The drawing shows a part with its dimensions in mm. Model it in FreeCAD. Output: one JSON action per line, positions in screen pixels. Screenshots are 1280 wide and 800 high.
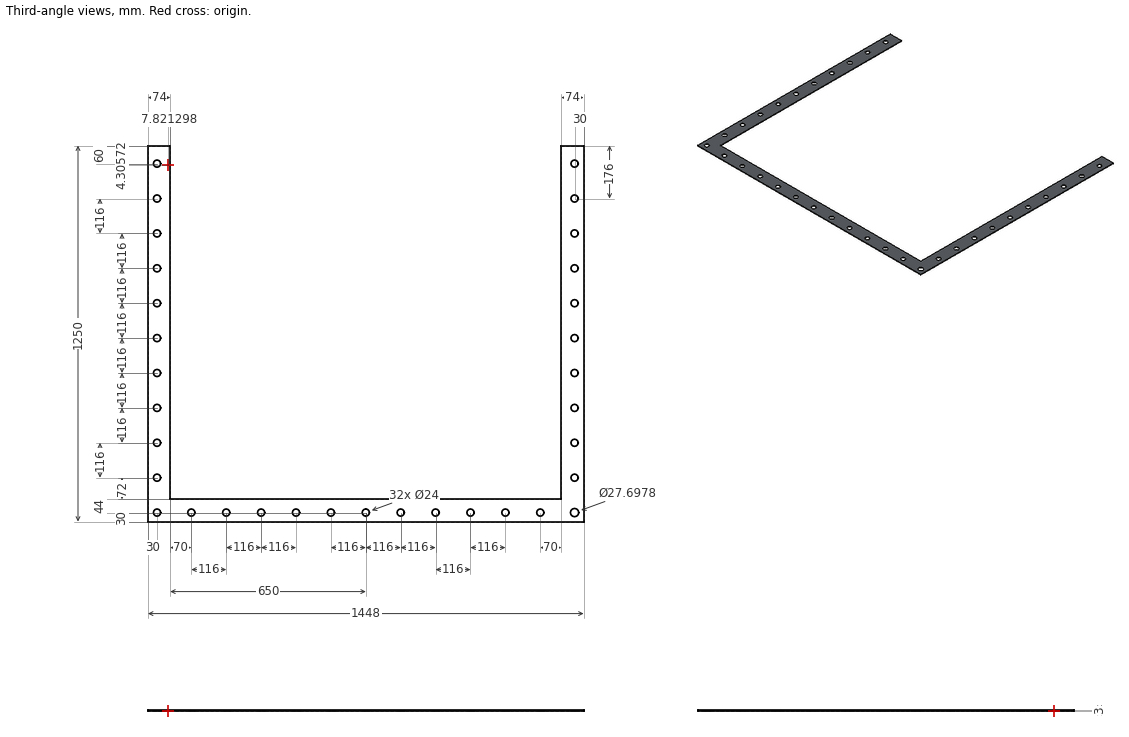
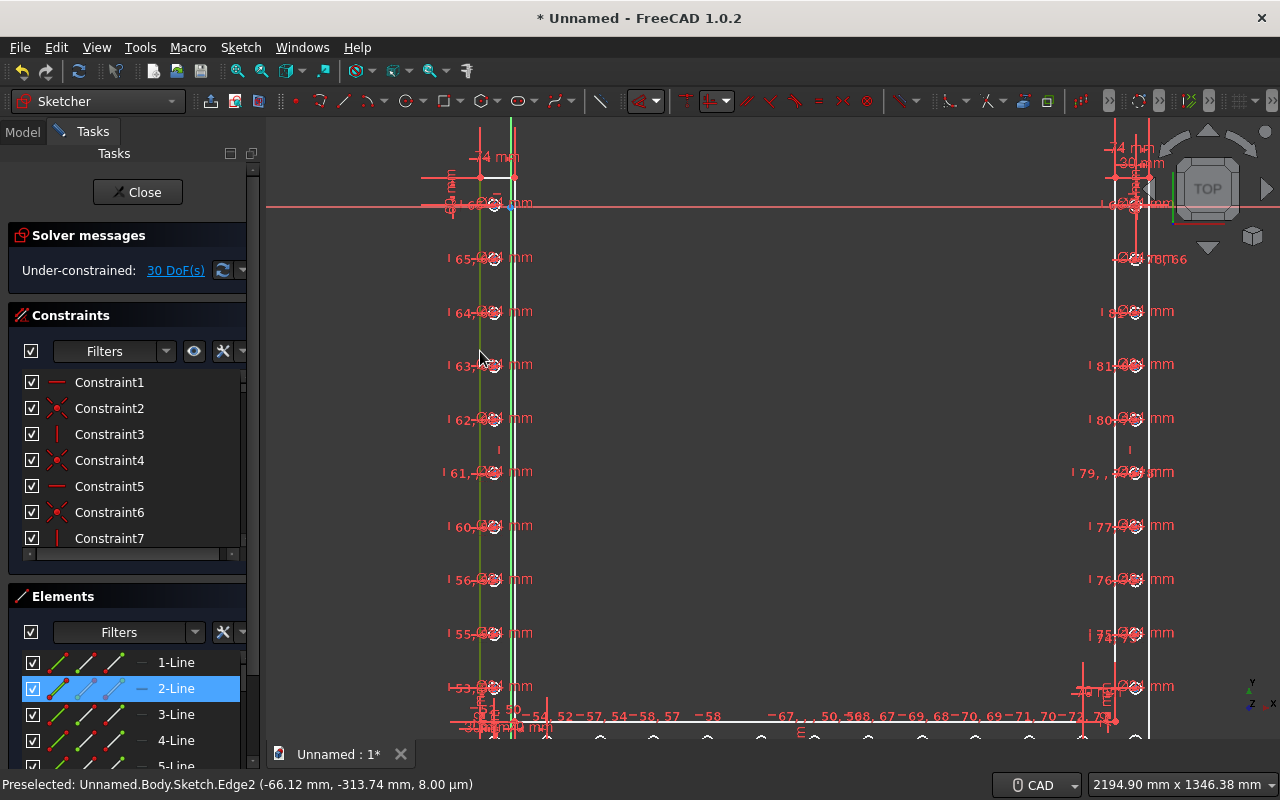
{"action": "left_click", "coordinate": [658, 102]}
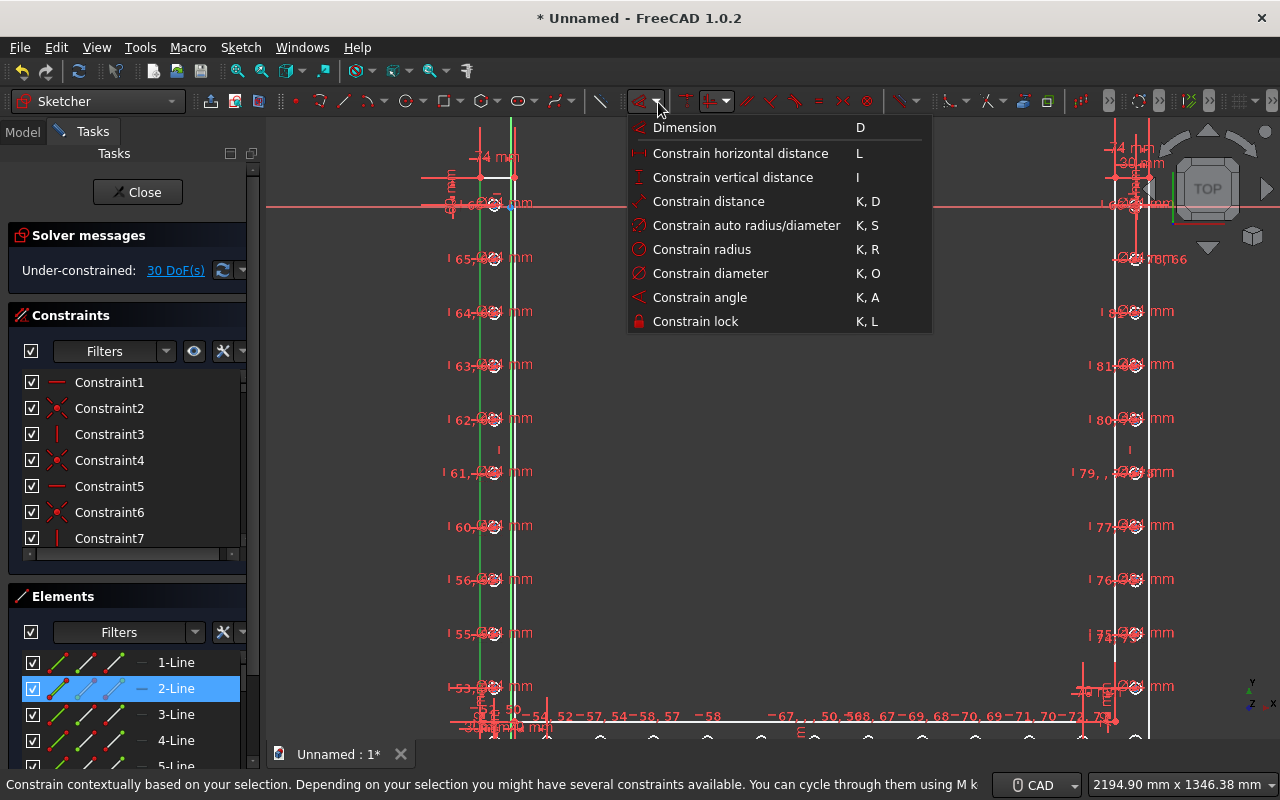
{"action": "left_click", "coordinate": [780, 177]}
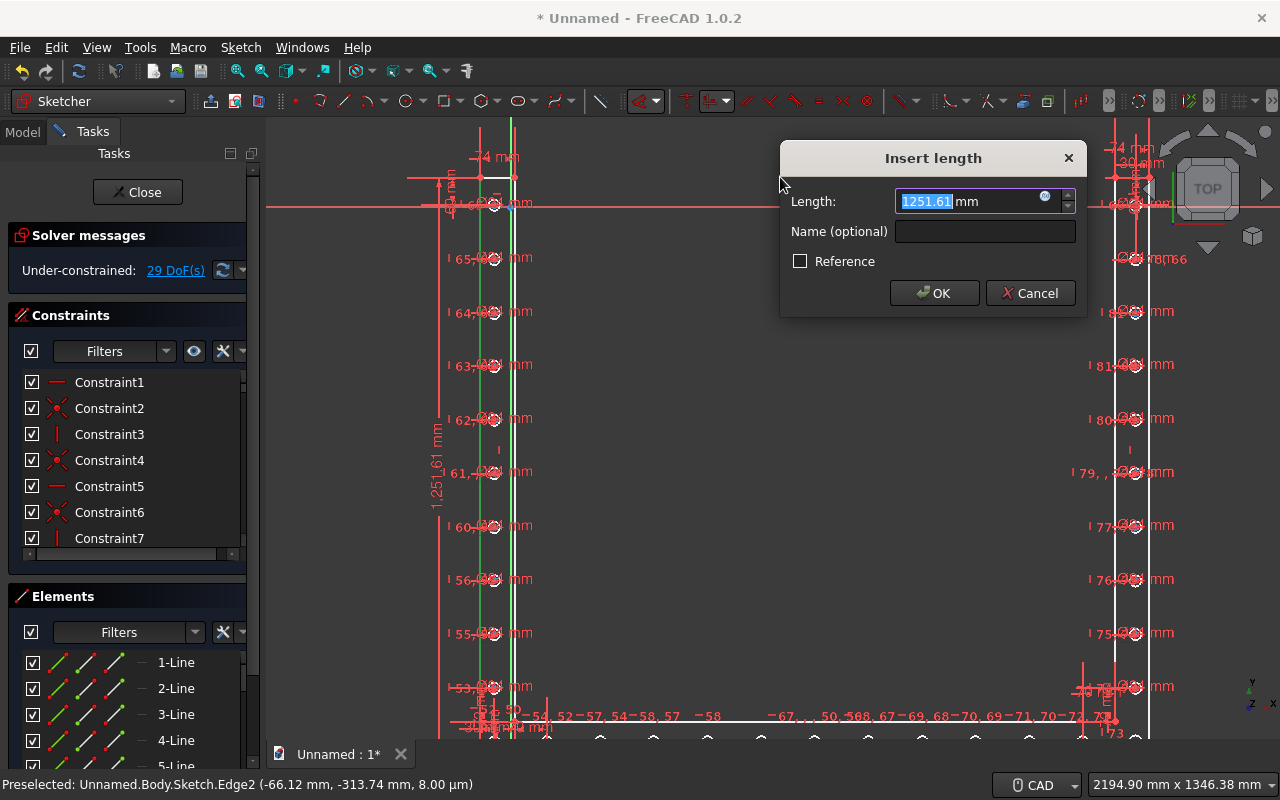
{"action": "type", "text": "1250"}
{"action": "key", "text": "Return"}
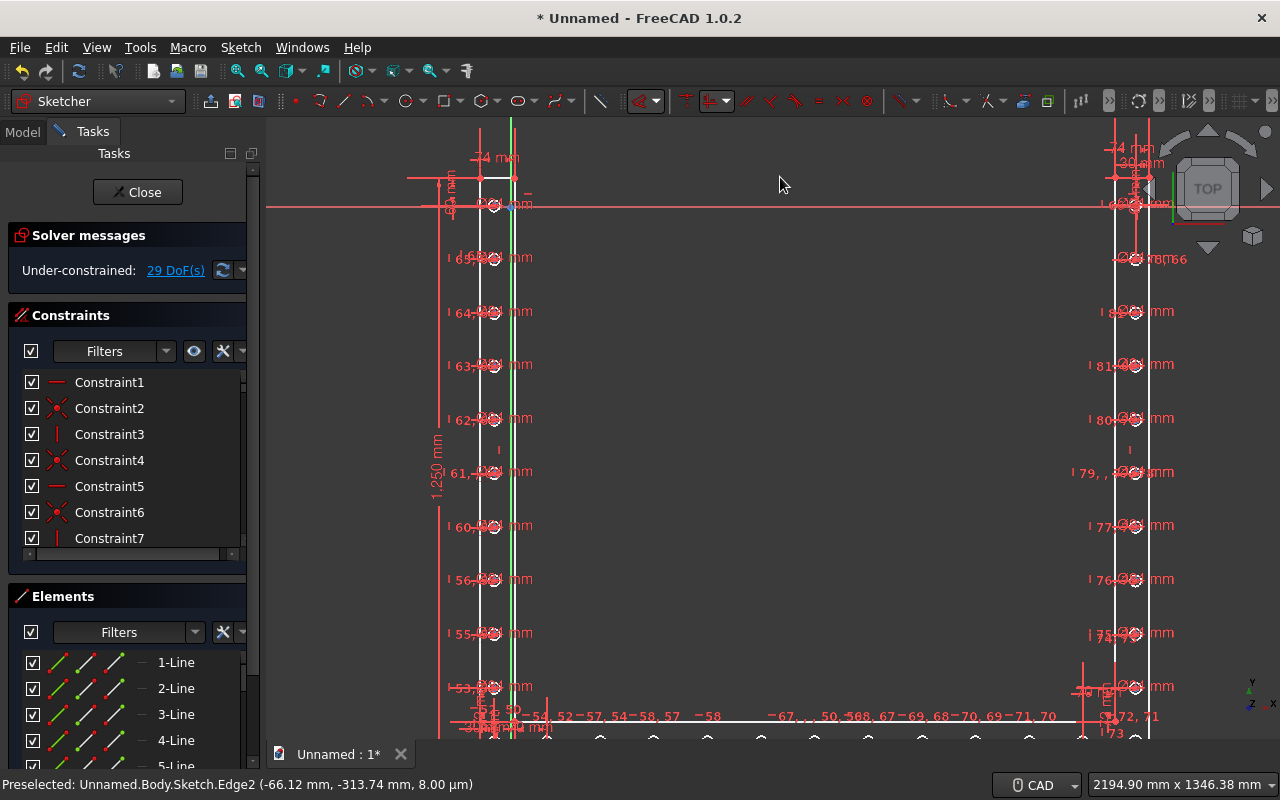
{"action": "scroll", "coordinate": [480, 351], "scroll_direction": "down", "scroll_amount": 2}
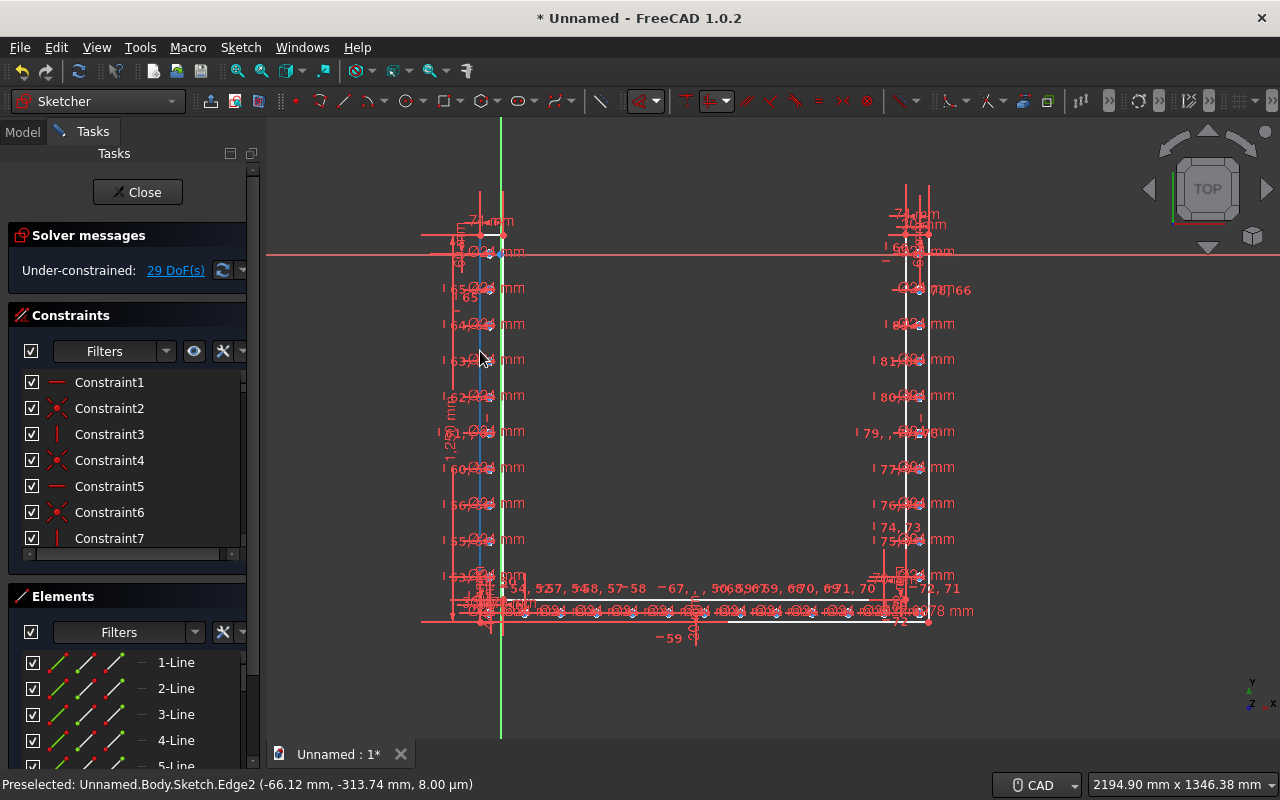
{"action": "left_click", "coordinate": [615, 622]}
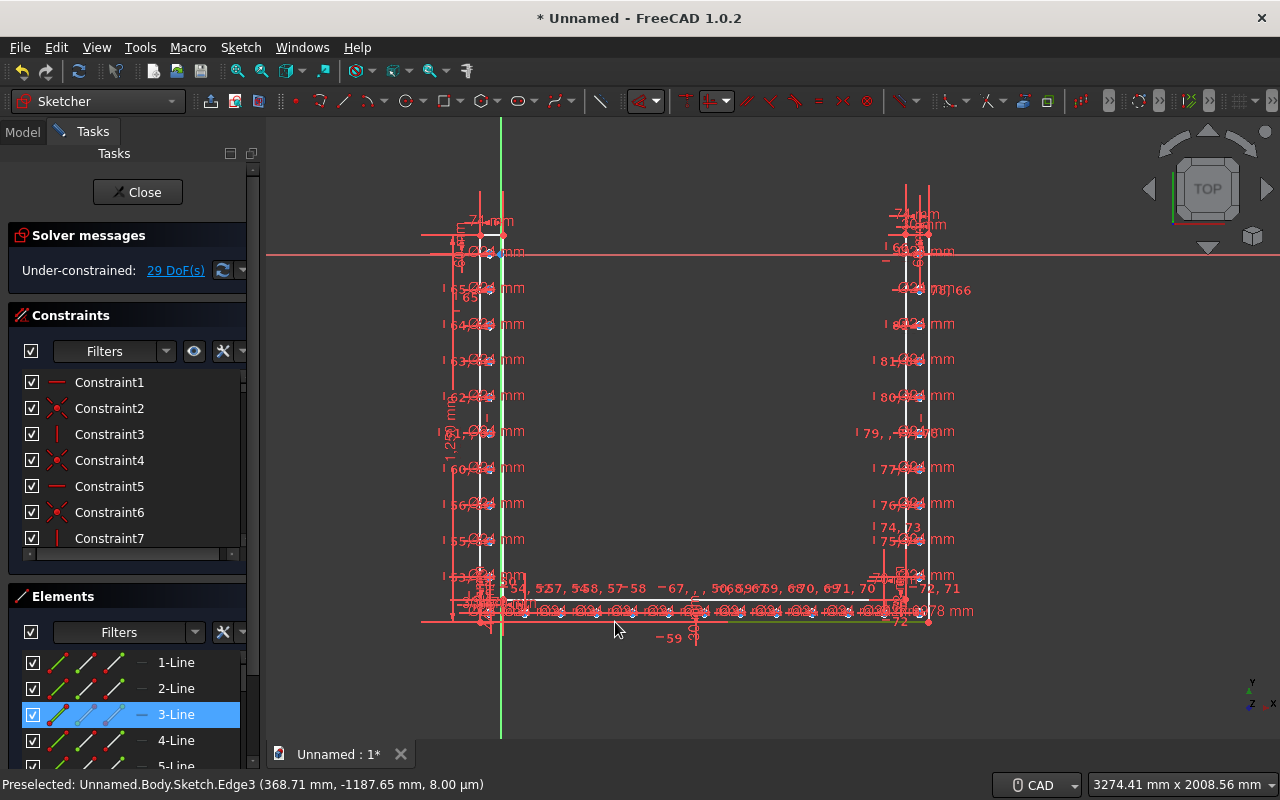
{"action": "left_click", "coordinate": [658, 102]}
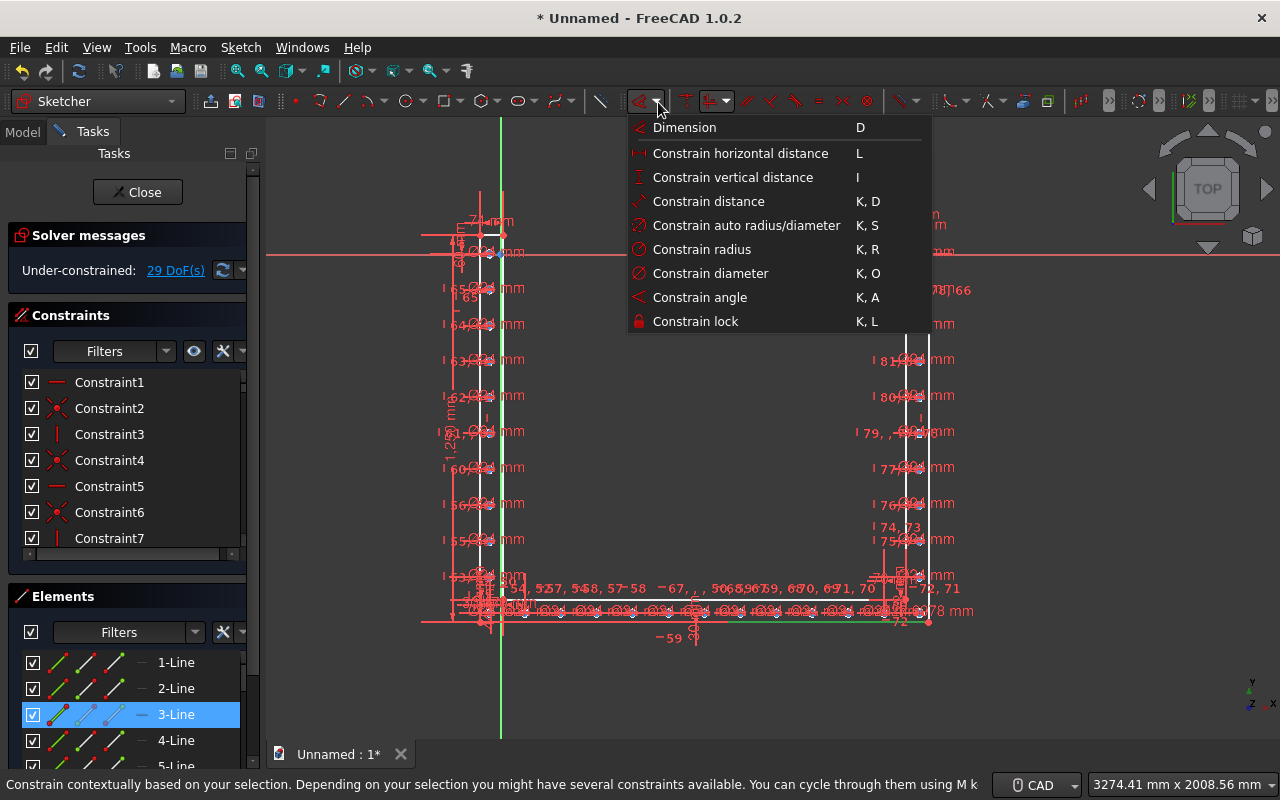
{"action": "left_click", "coordinate": [780, 153]}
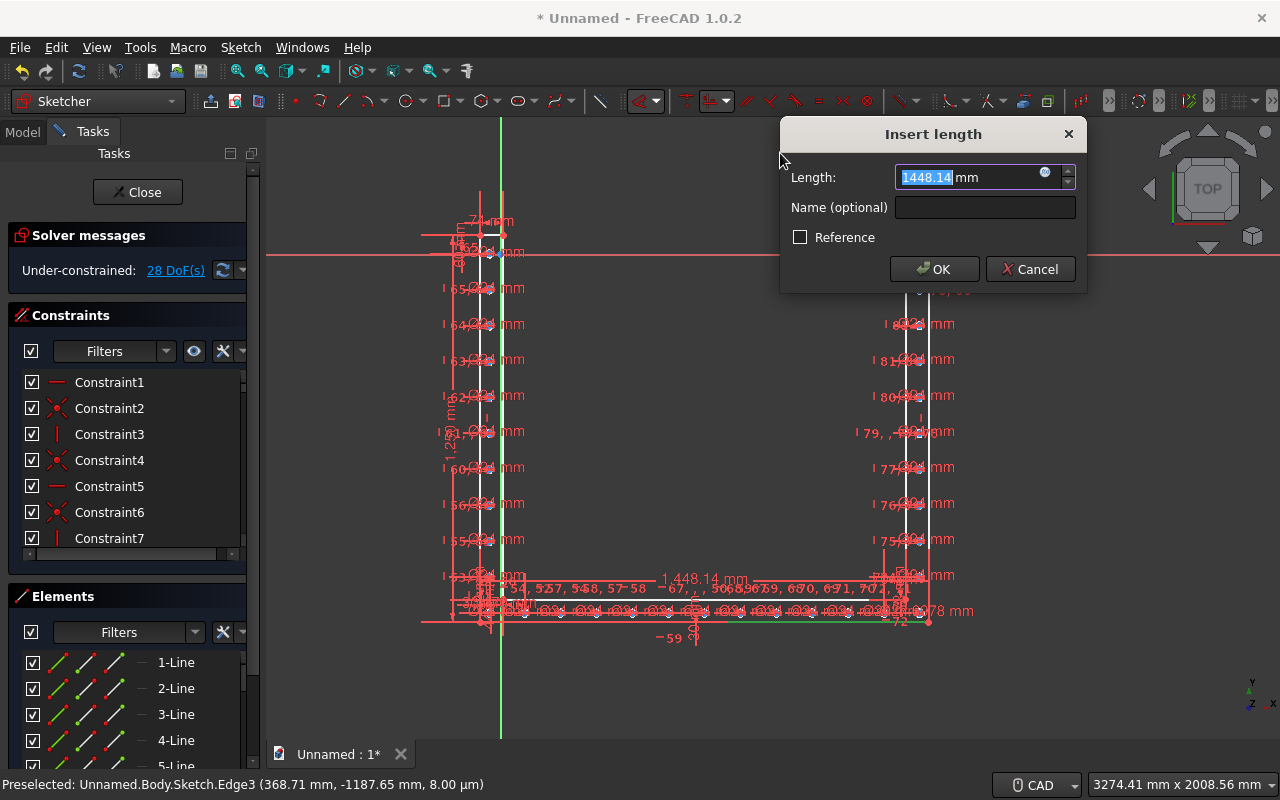
{"action": "type", "text": "1448"}
{"action": "key", "text": "Return"}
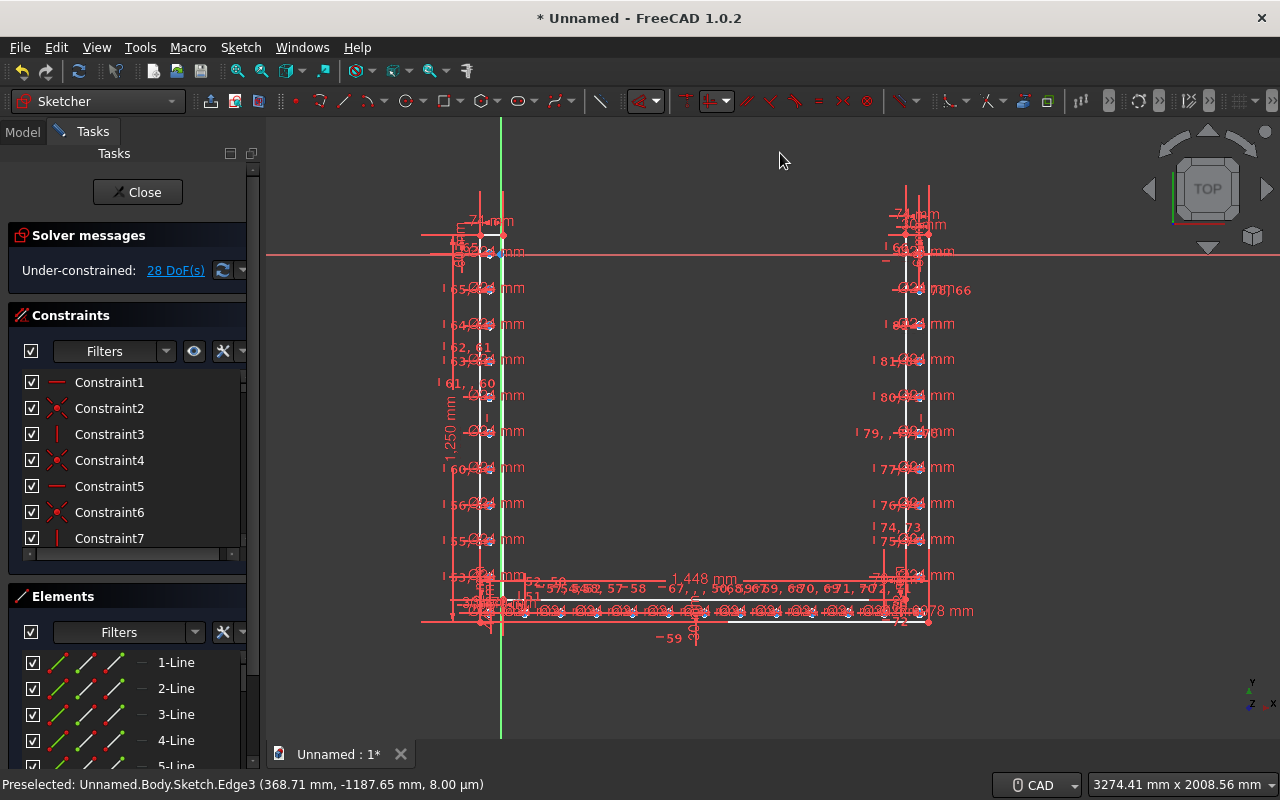
{"action": "scroll", "coordinate": [929, 351], "scroll_direction": "up", "scroll_amount": 2}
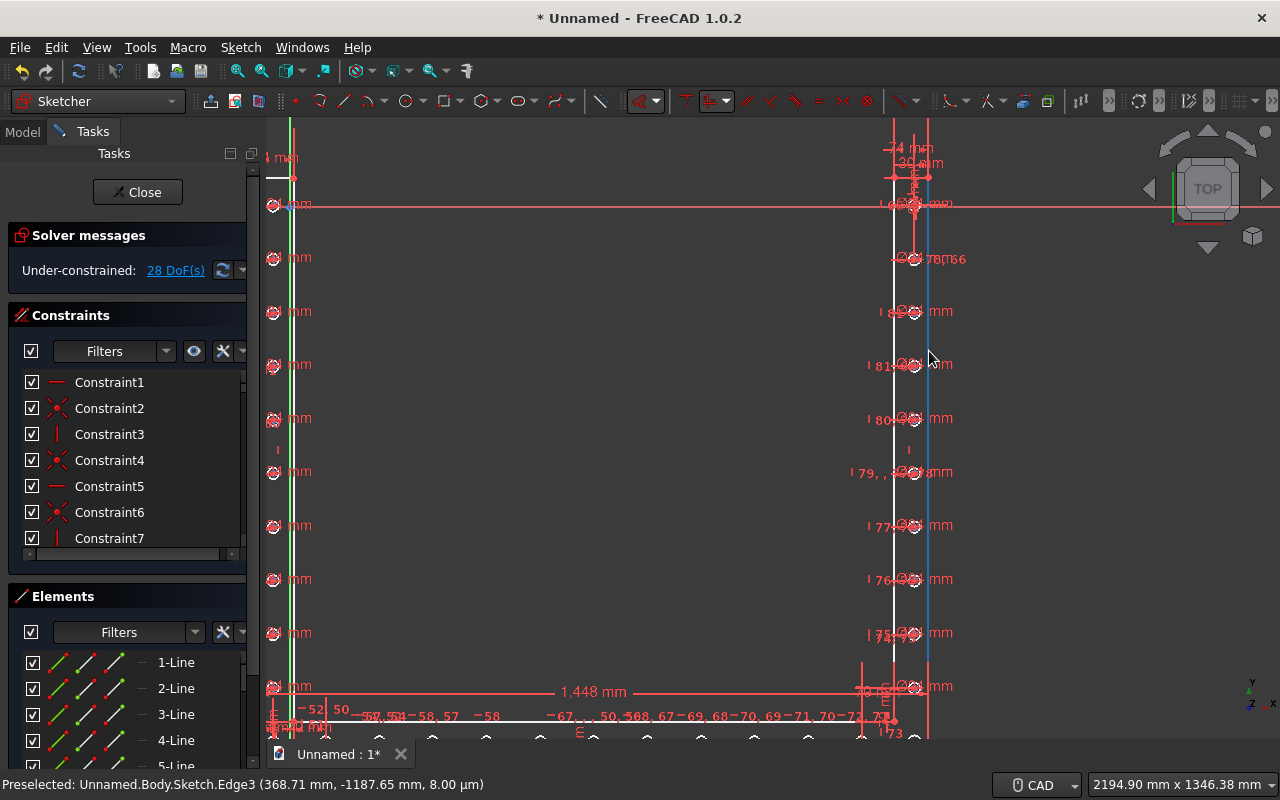
{"action": "left_click", "coordinate": [928, 351]}